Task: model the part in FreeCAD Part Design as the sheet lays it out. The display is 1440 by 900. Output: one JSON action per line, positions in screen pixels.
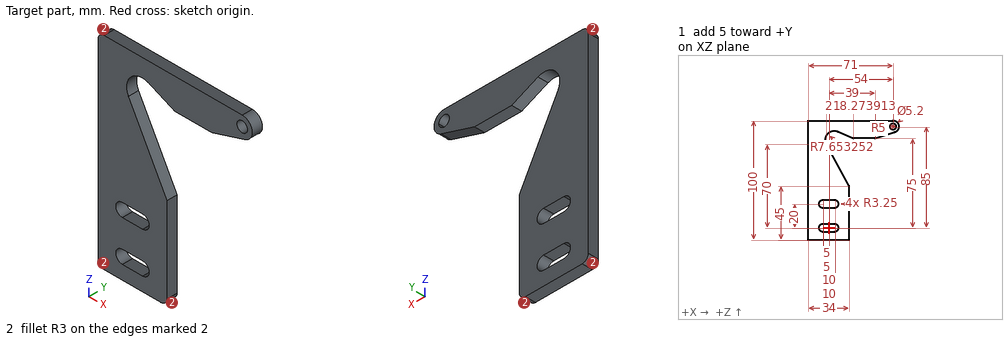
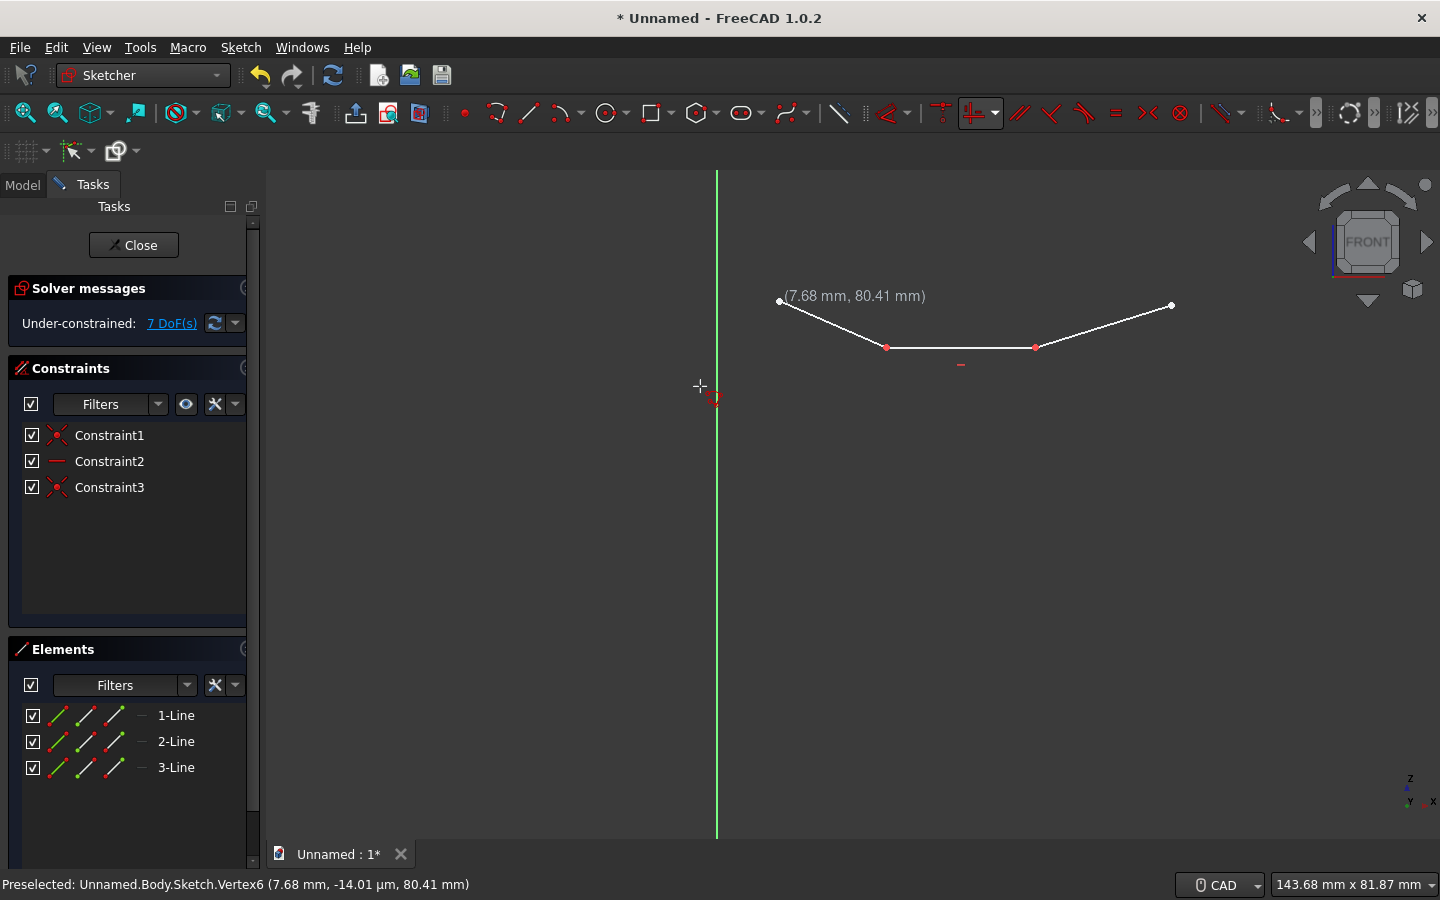
{"action": "left_click", "coordinate": [701, 386]}
{"action": "left_click", "coordinate": [856, 672]}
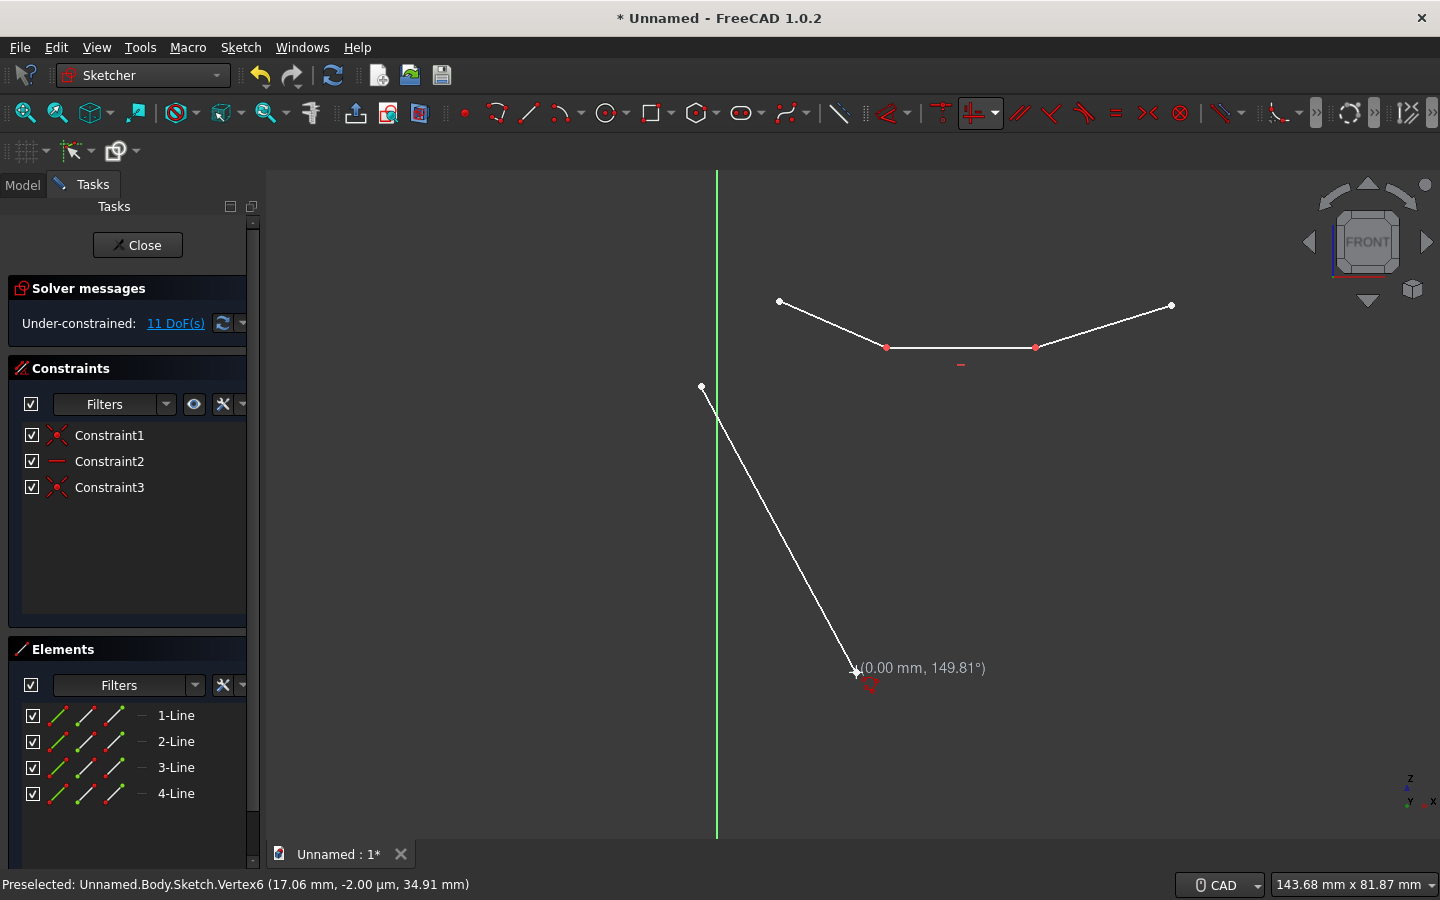
{"action": "scroll", "coordinate": [658, 350], "scroll_direction": "down", "scroll_amount": 3}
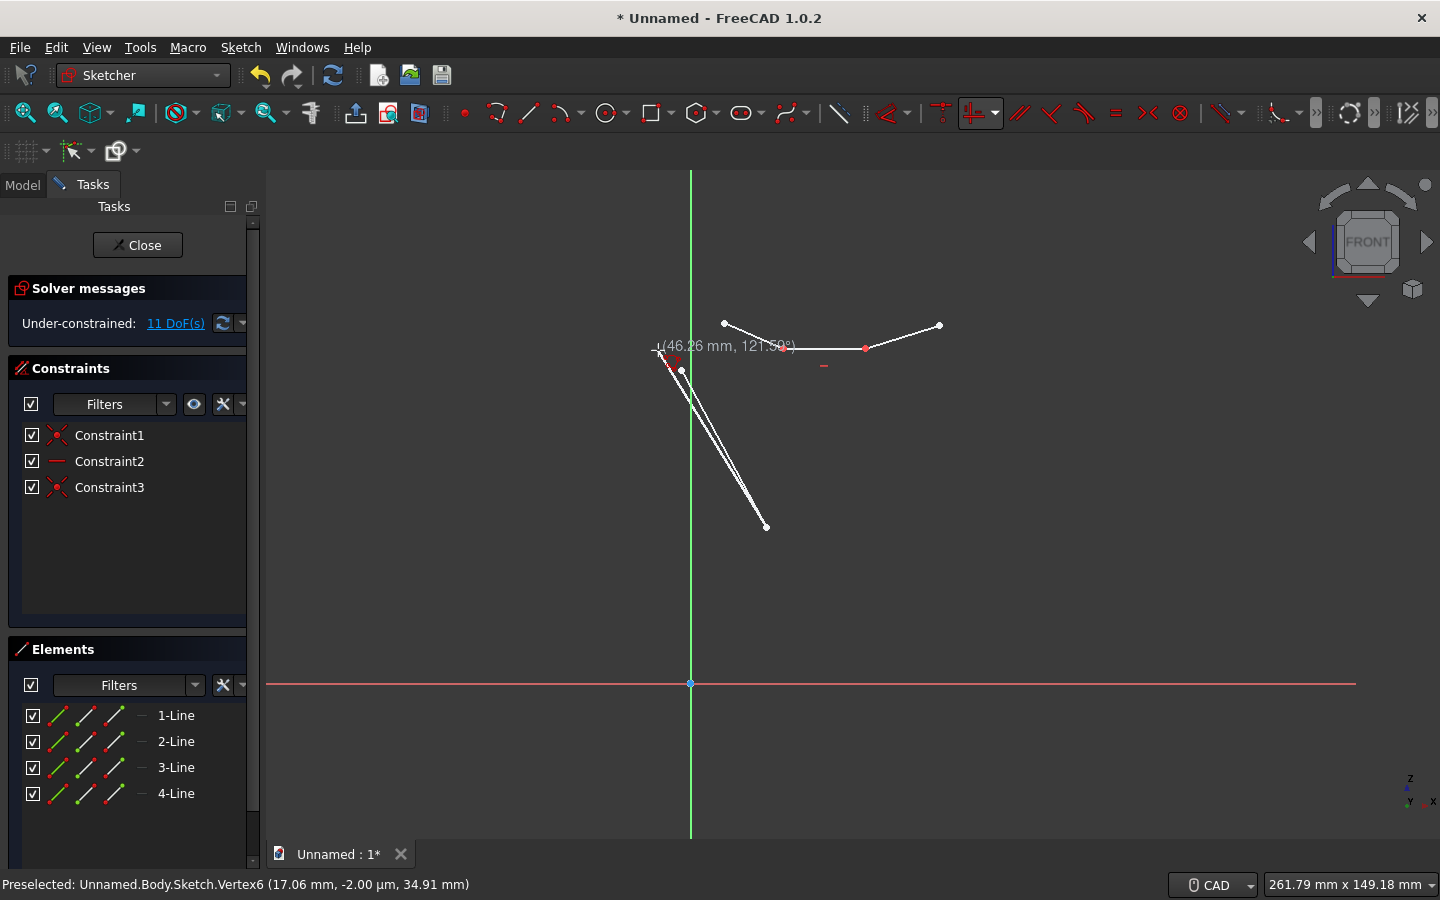
{"action": "left_click", "coordinate": [767, 729]}
{"action": "left_click", "coordinate": [614, 729]}
{"action": "left_click", "coordinate": [614, 280]}
{"action": "left_click", "coordinate": [933, 280]}
{"action": "right_click", "coordinate": [933, 280]}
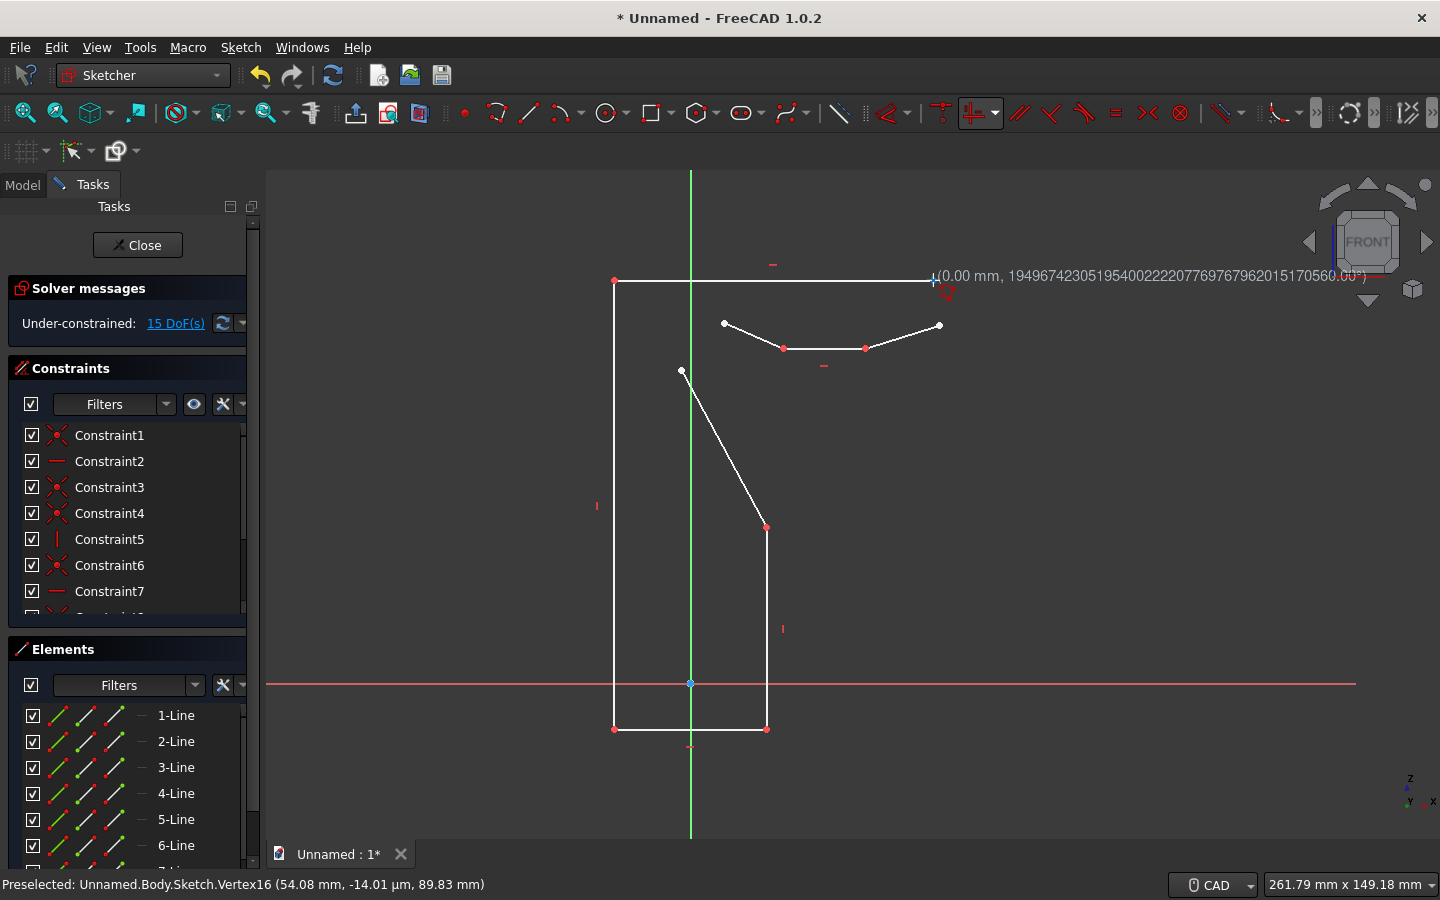
{"action": "left_click", "coordinate": [584, 114]}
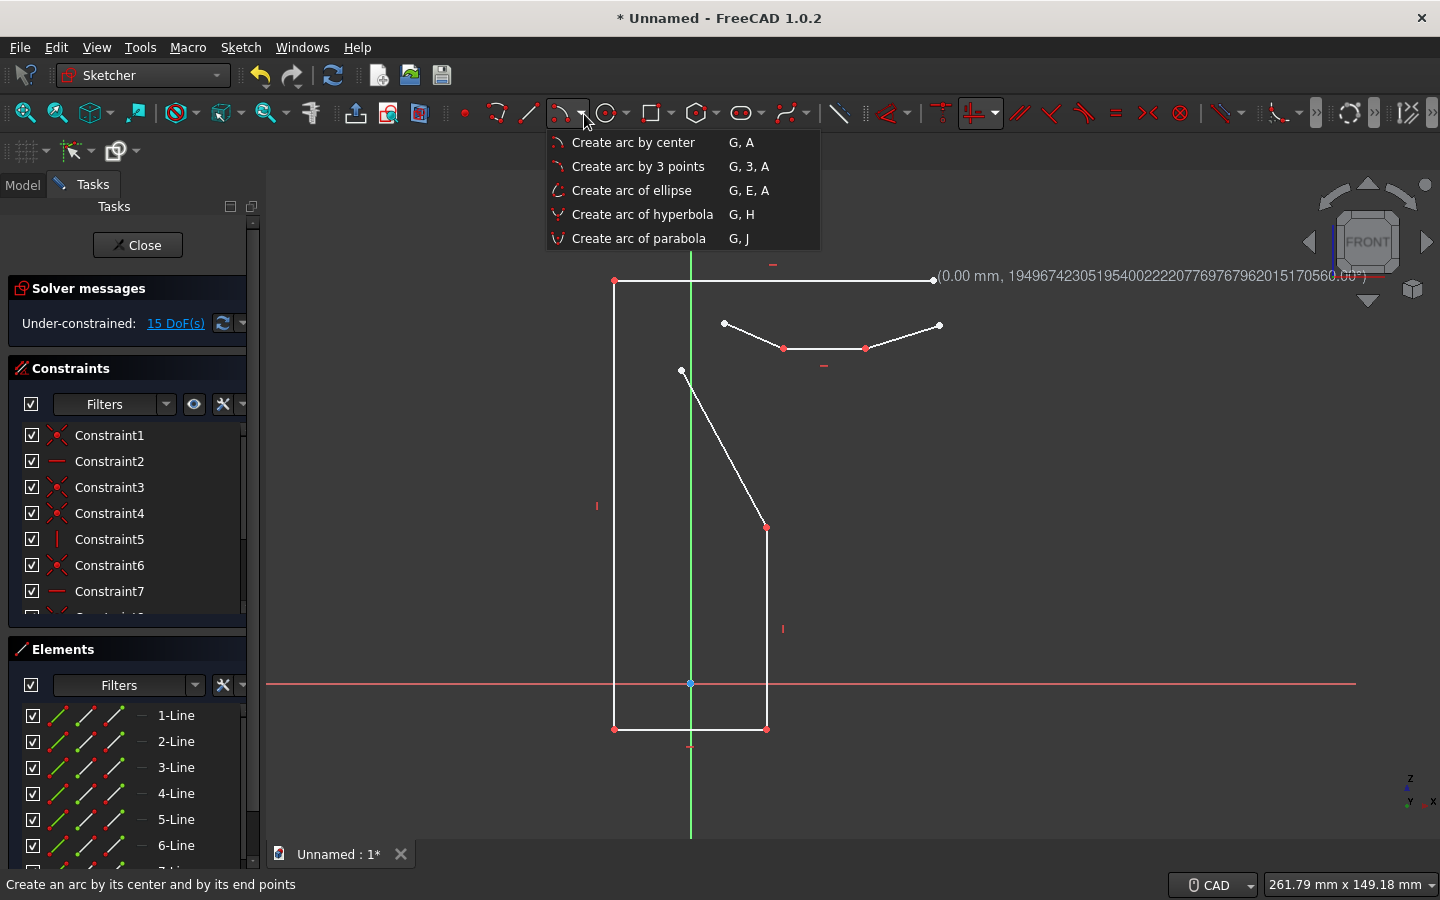
{"action": "left_click", "coordinate": [684, 166]}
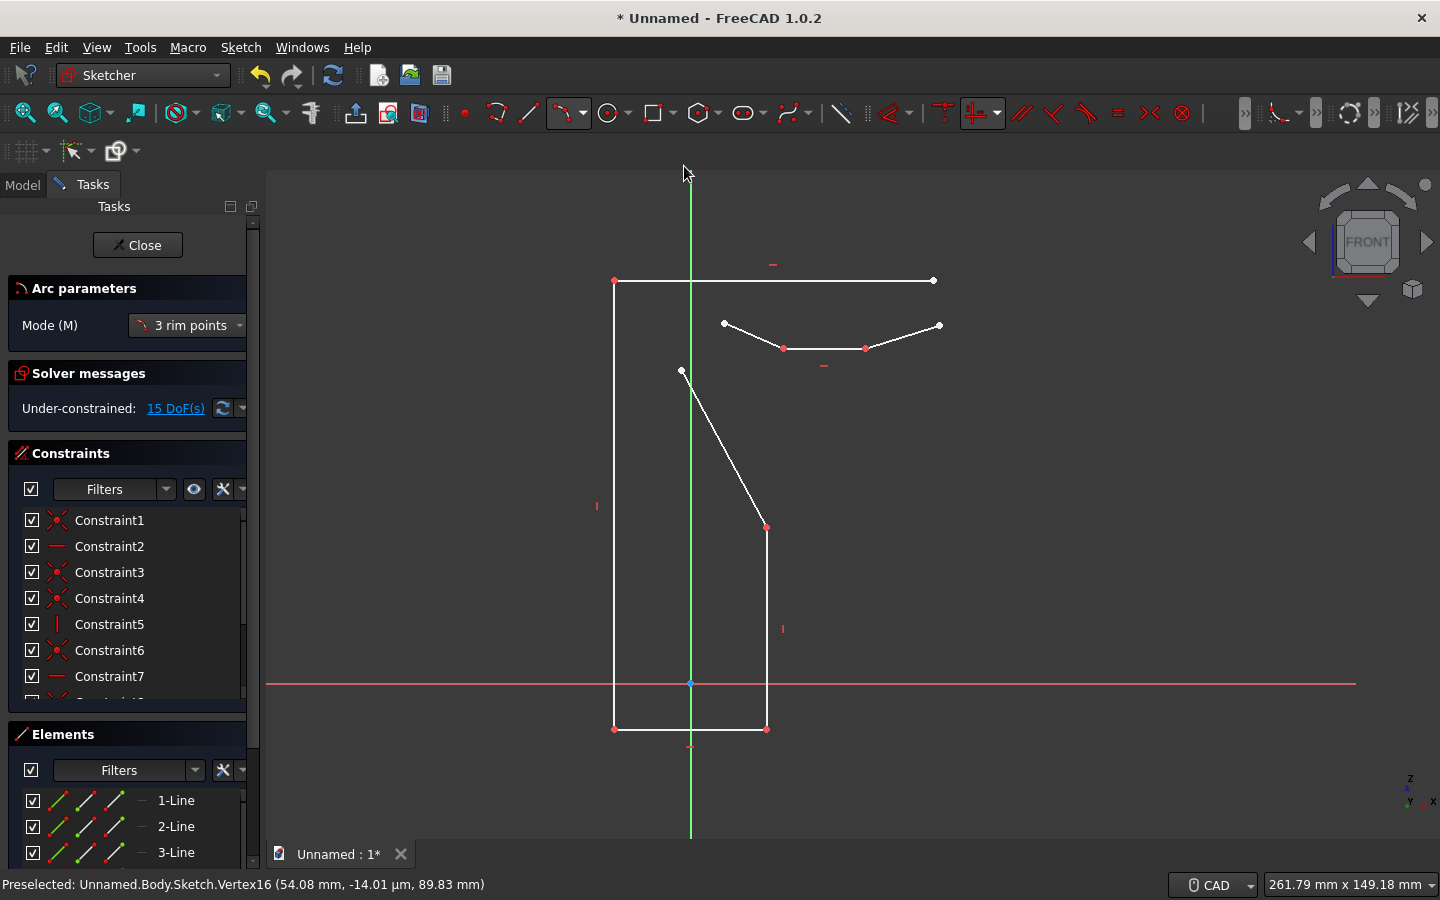
{"action": "left_click", "coordinate": [725, 323]}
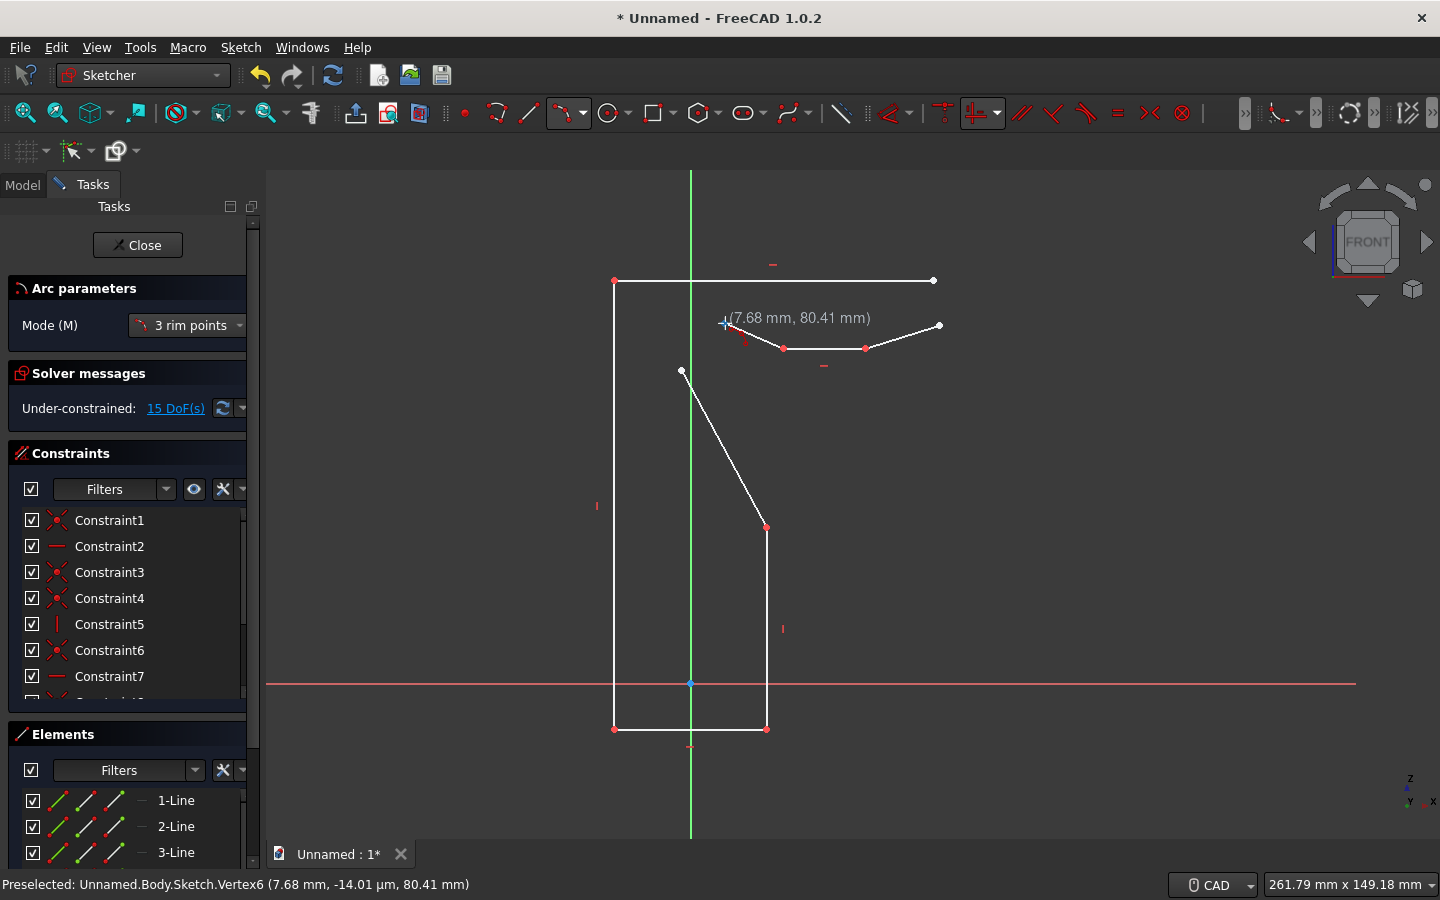
{"action": "scroll", "coordinate": [682, 370], "scroll_direction": "up", "scroll_amount": 3}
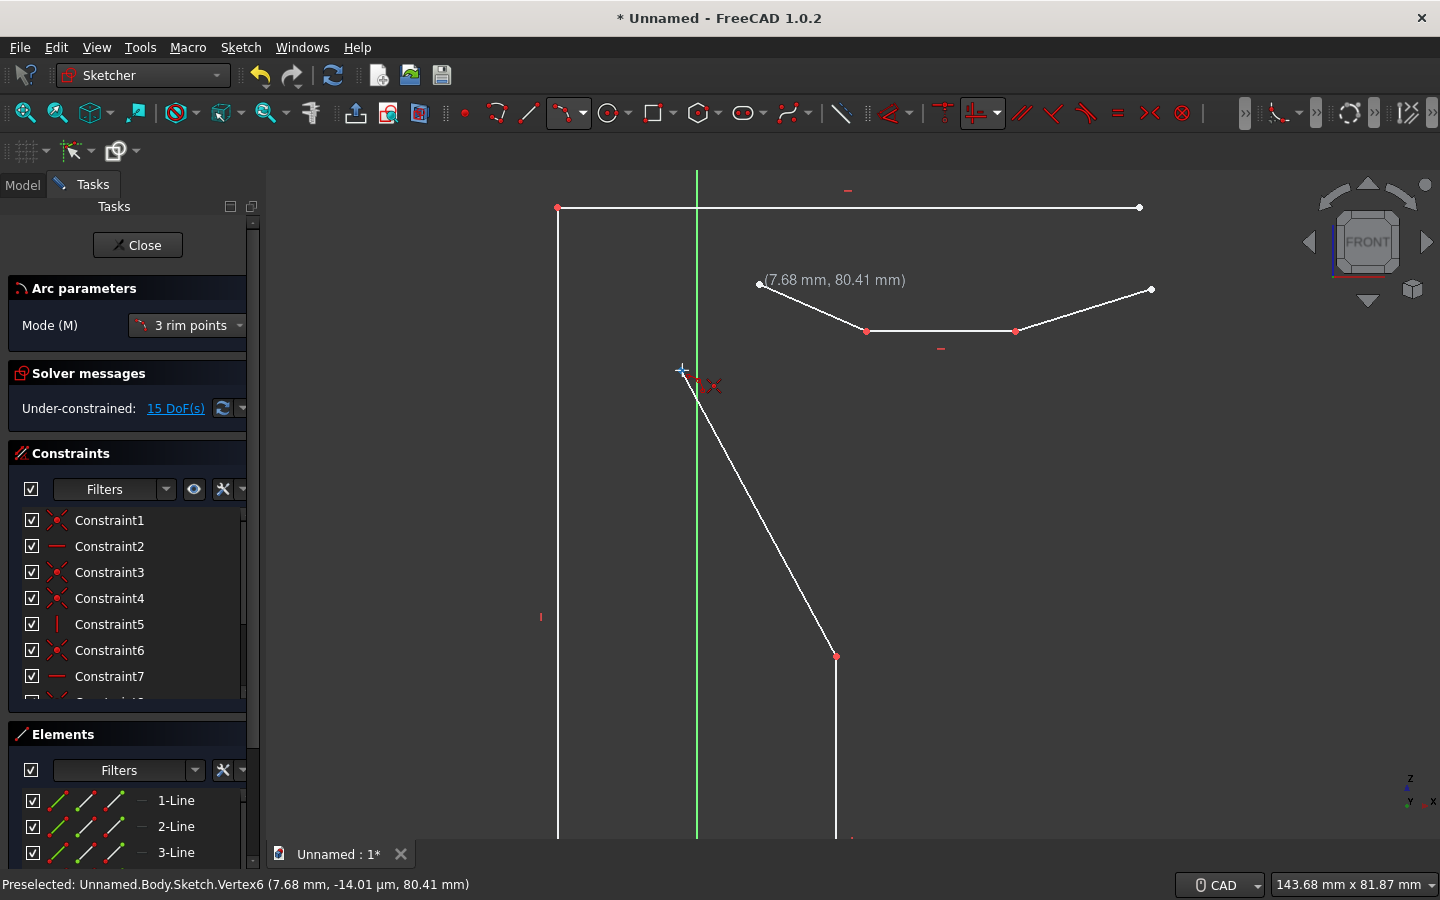
{"action": "left_click", "coordinate": [681, 371]}
{"action": "left_click", "coordinate": [675, 324]}